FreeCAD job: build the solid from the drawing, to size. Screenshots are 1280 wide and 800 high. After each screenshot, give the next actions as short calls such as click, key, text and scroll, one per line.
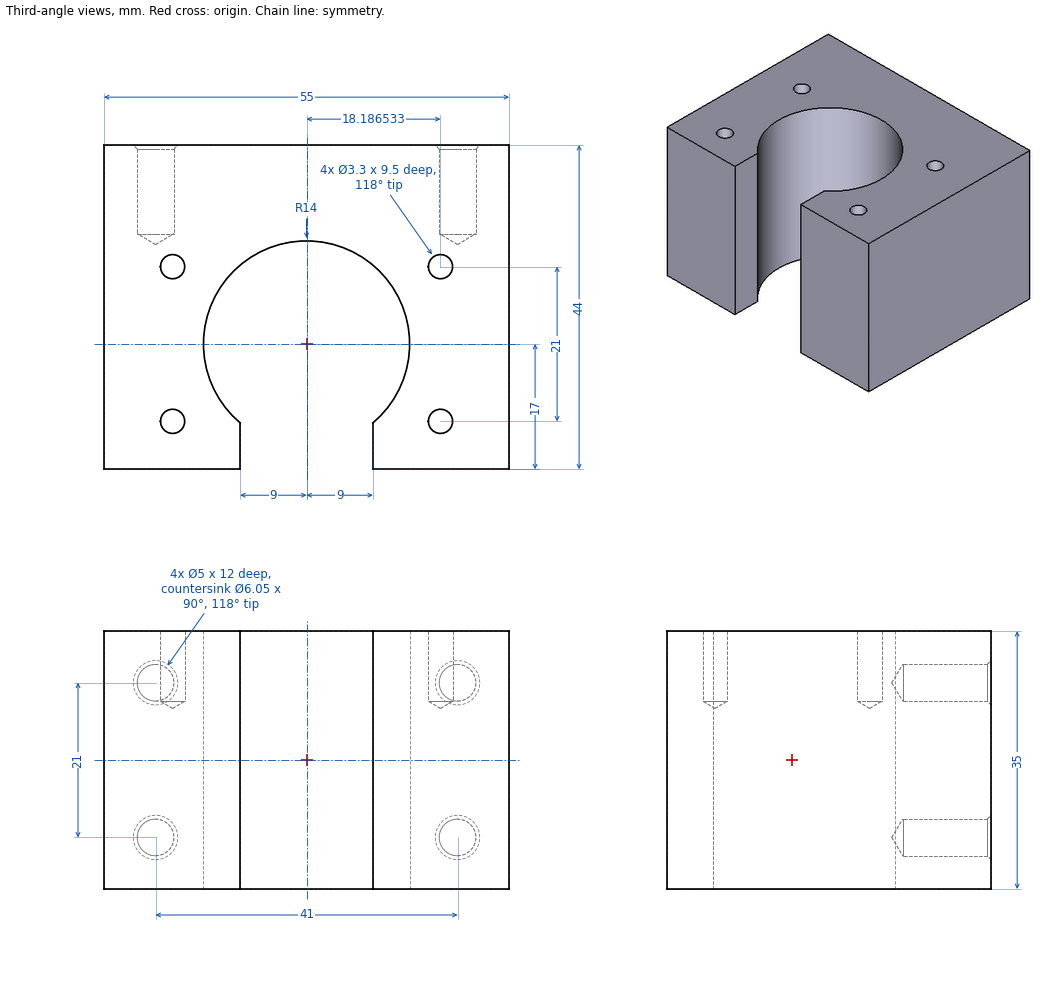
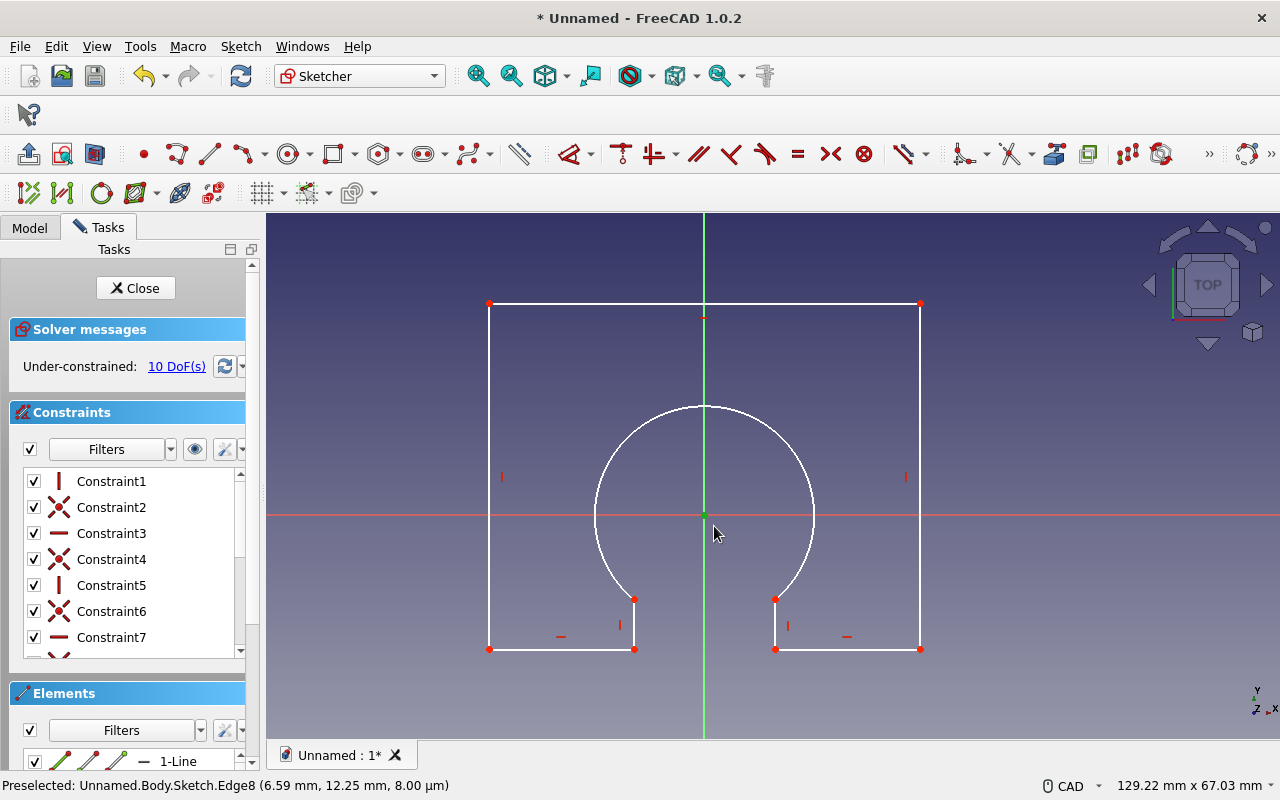
click(621, 154)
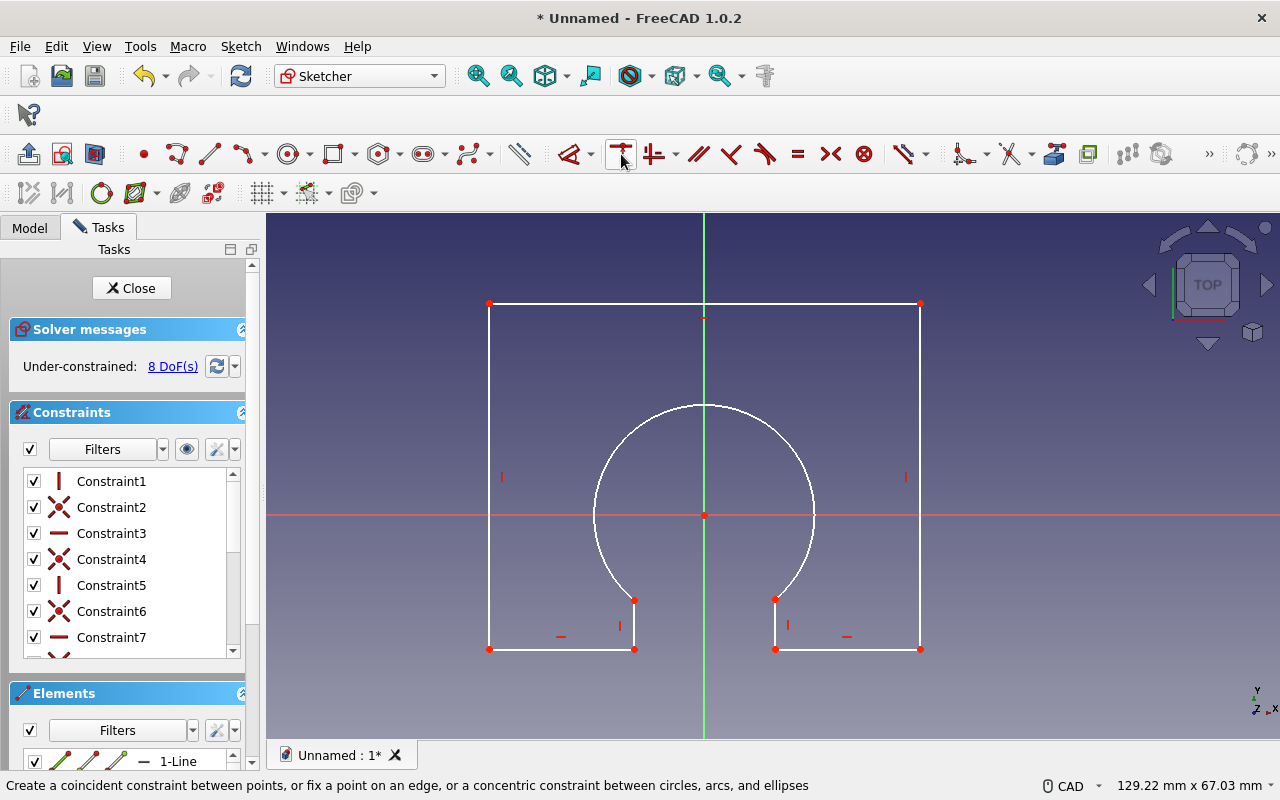
click(920, 650)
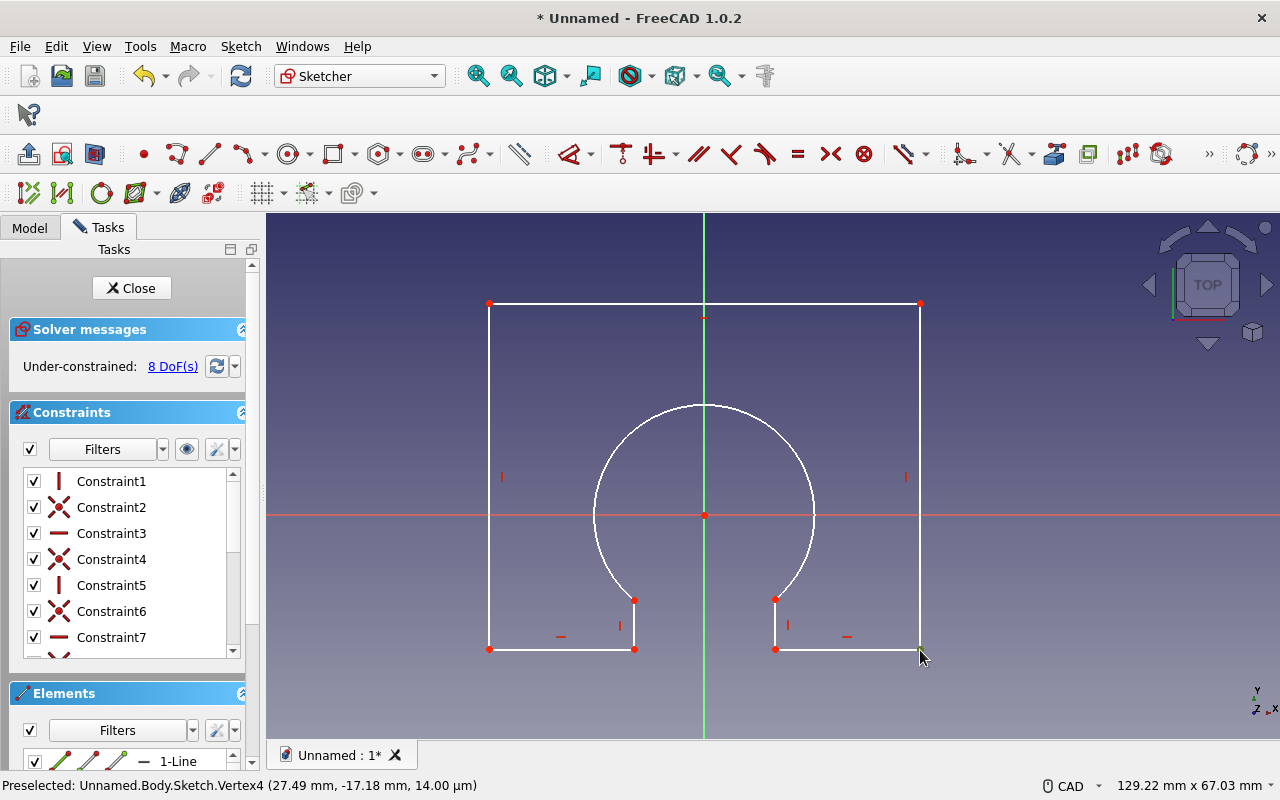
click(489, 650)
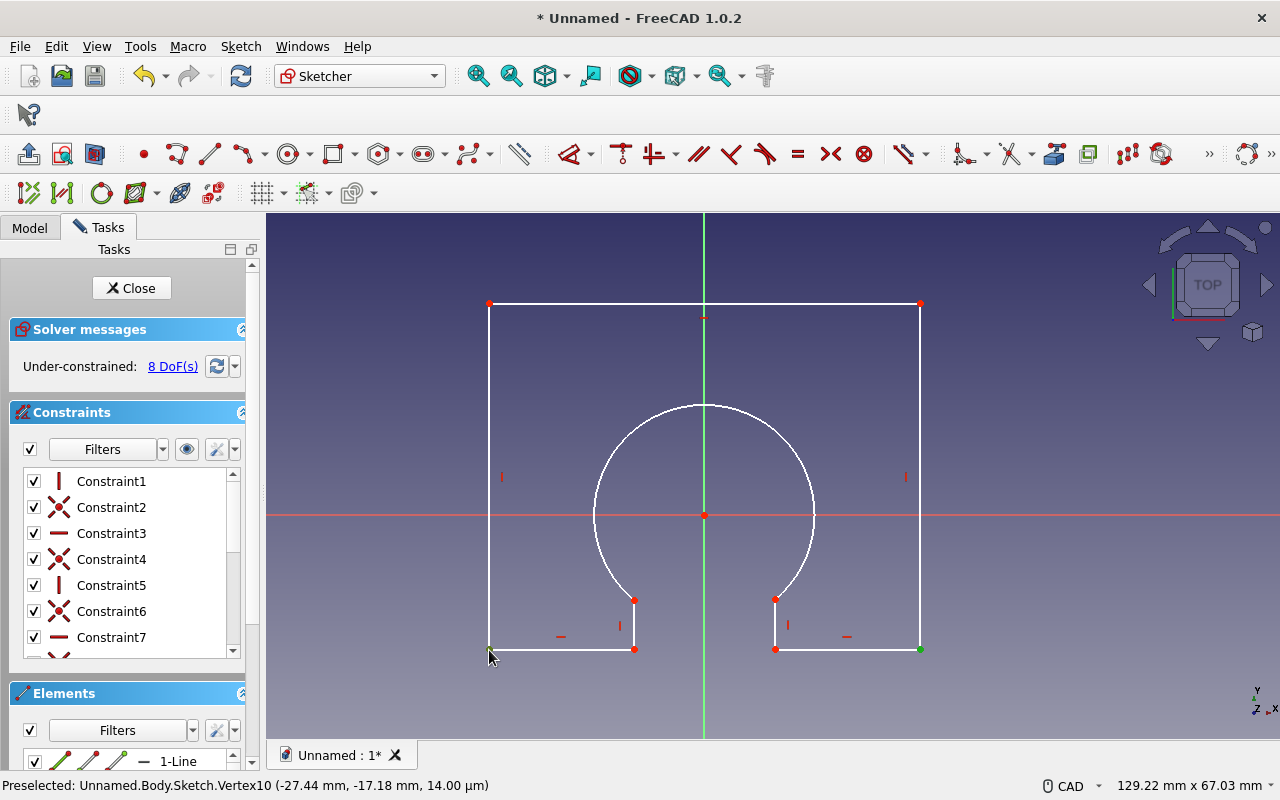
click(704, 677)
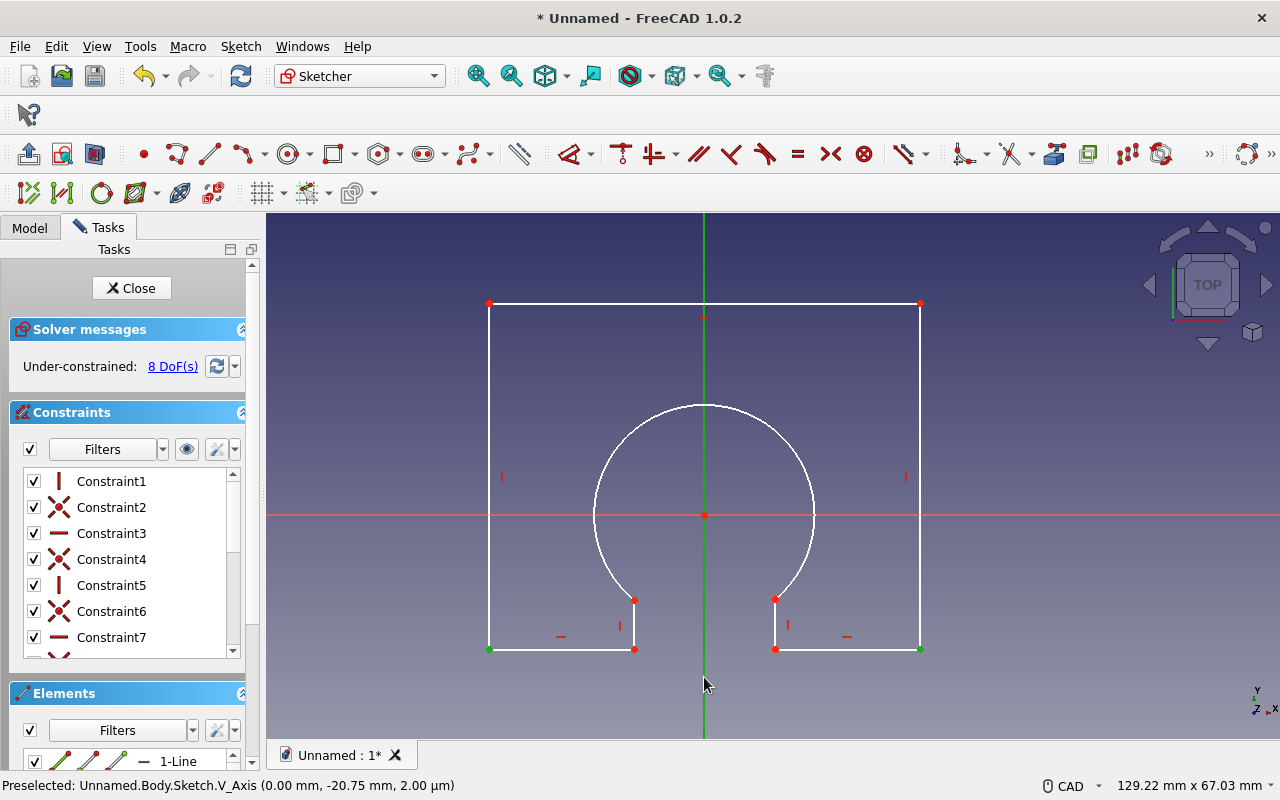
click(831, 154)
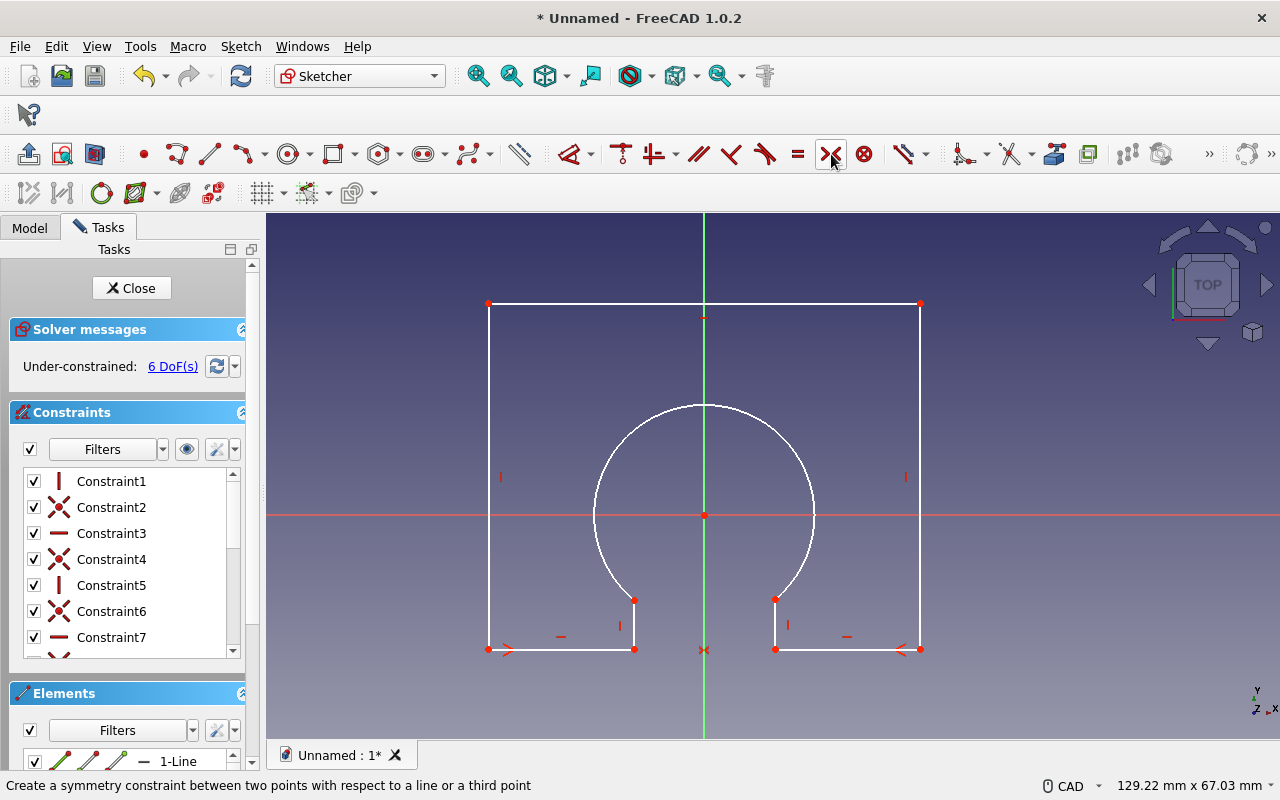
click(568, 154)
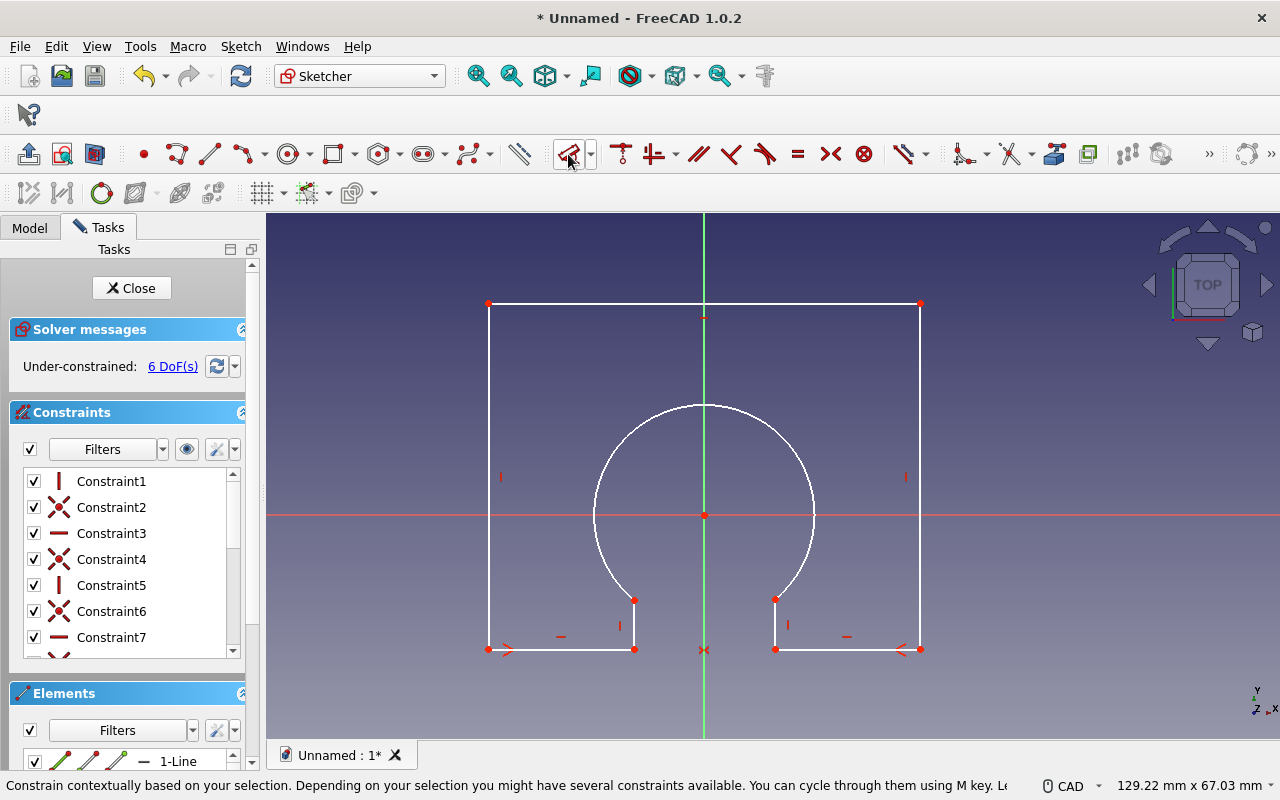
click(796, 453)
click(822, 435)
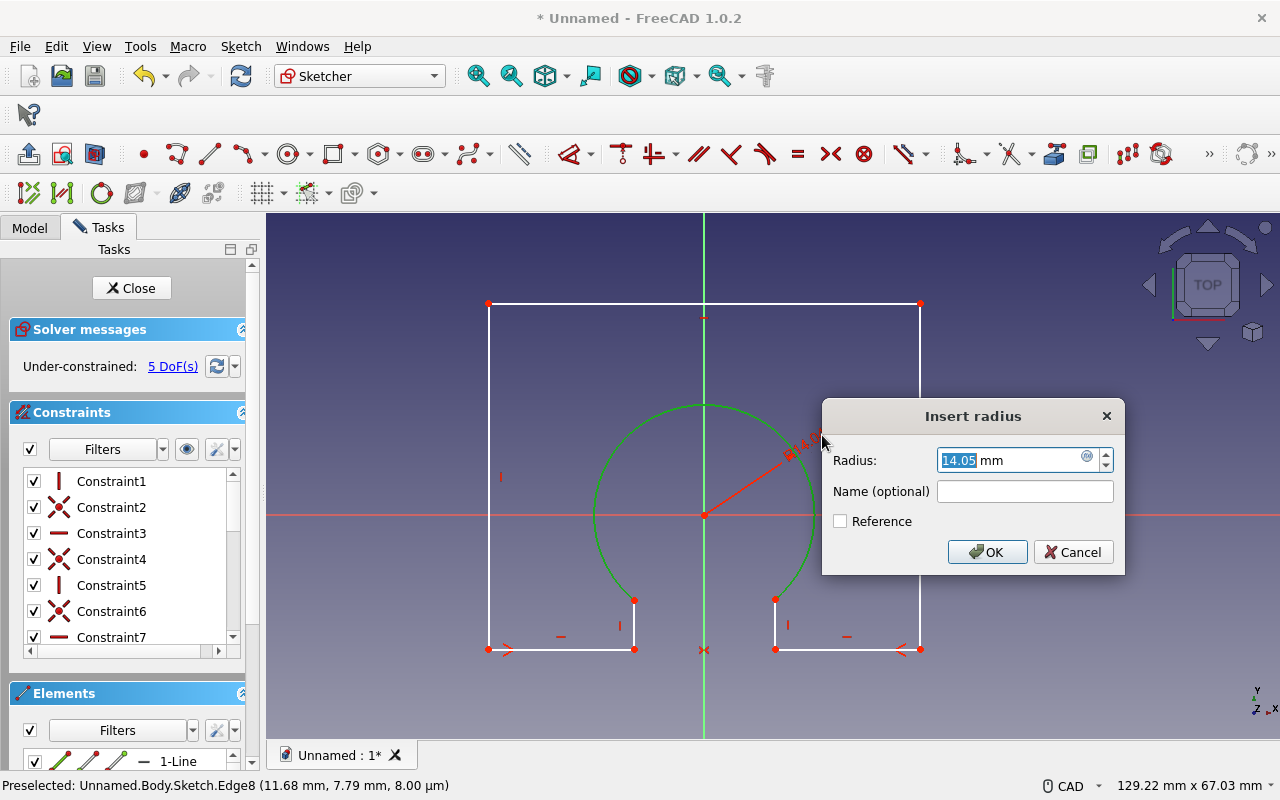
text(14)
key(Return)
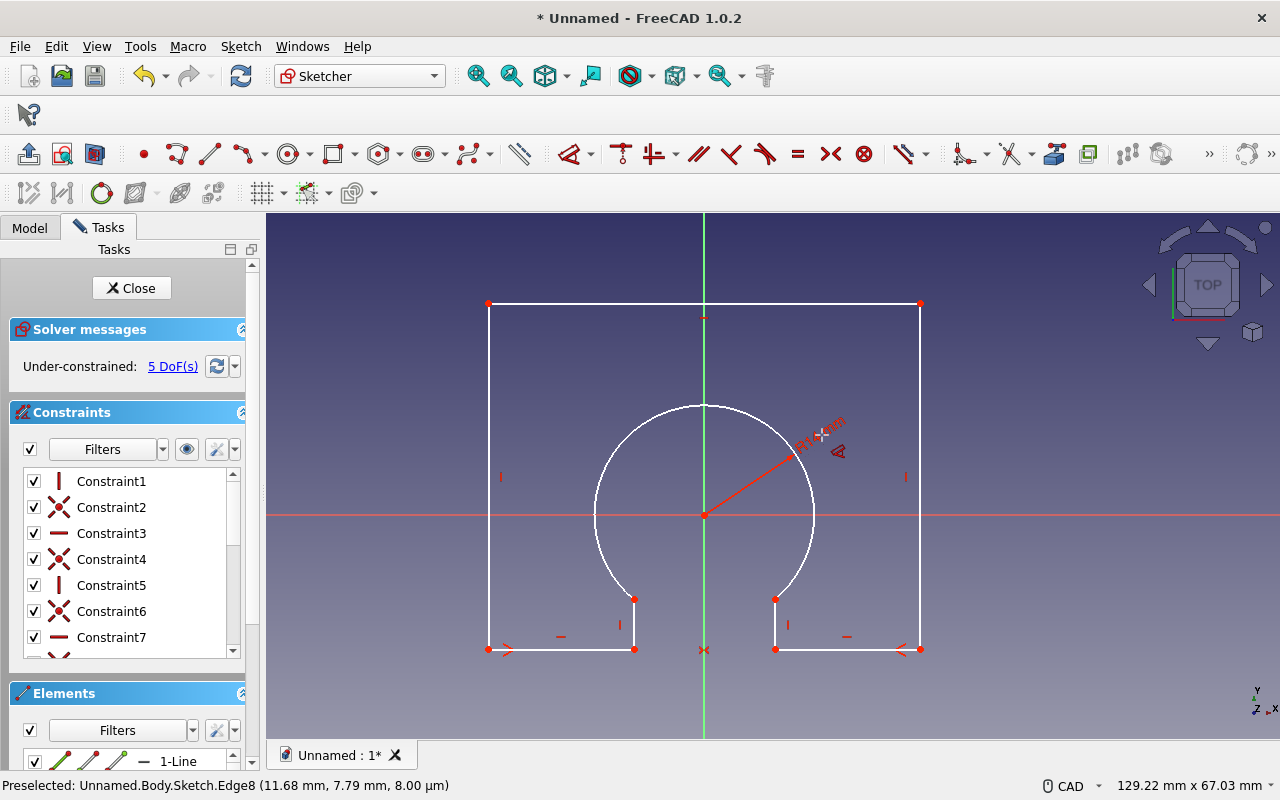
click(920, 546)
click(954, 477)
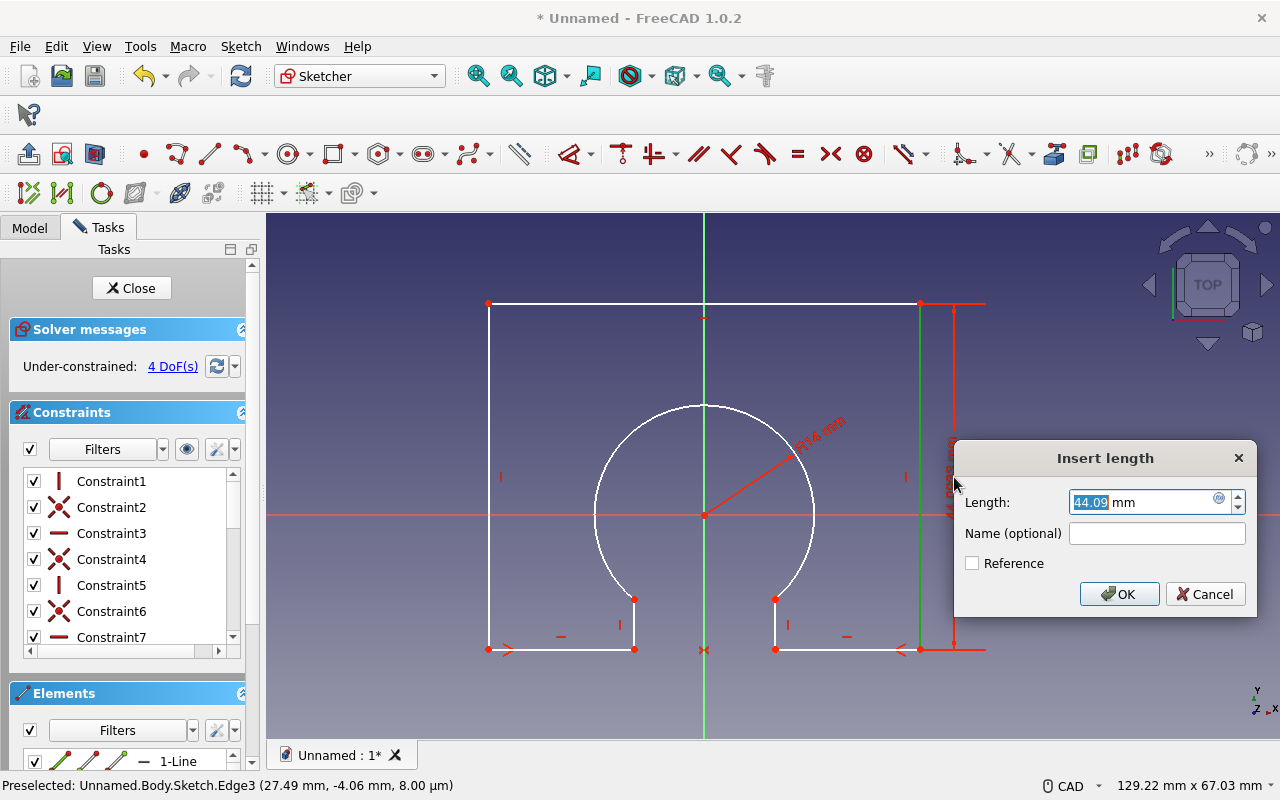
text(44)
key(Return)